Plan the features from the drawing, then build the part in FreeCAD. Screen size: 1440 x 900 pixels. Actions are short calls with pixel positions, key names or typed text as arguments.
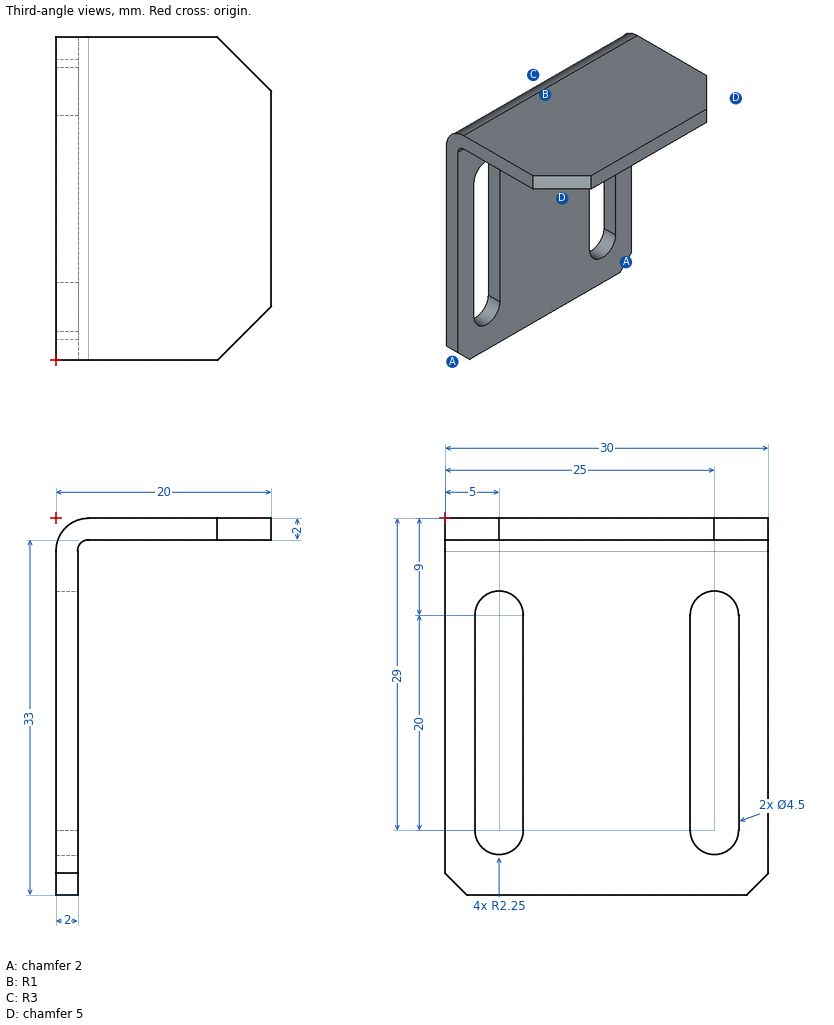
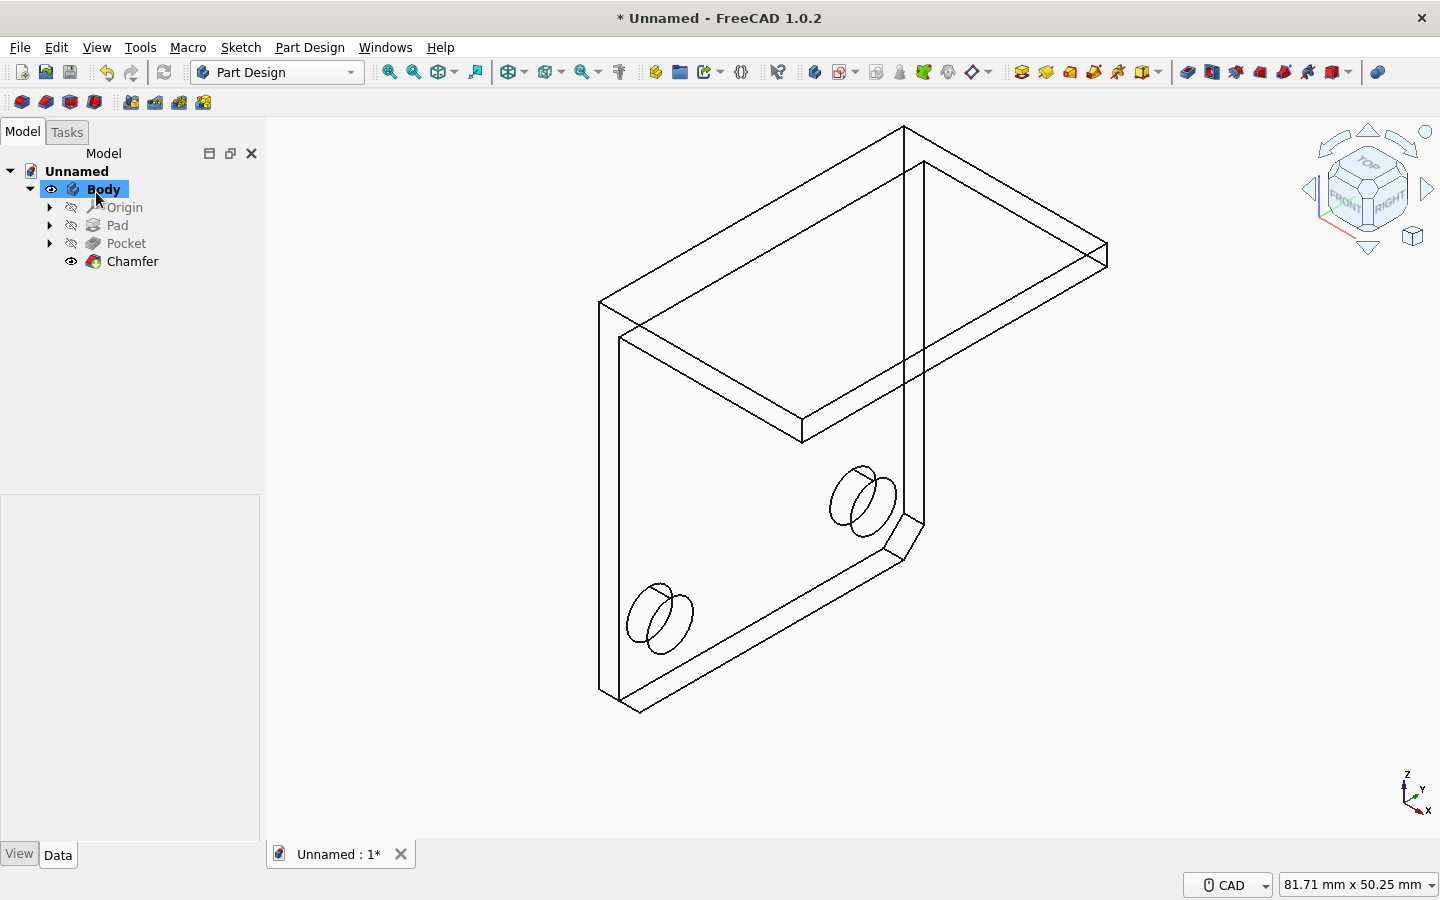
click(772, 248)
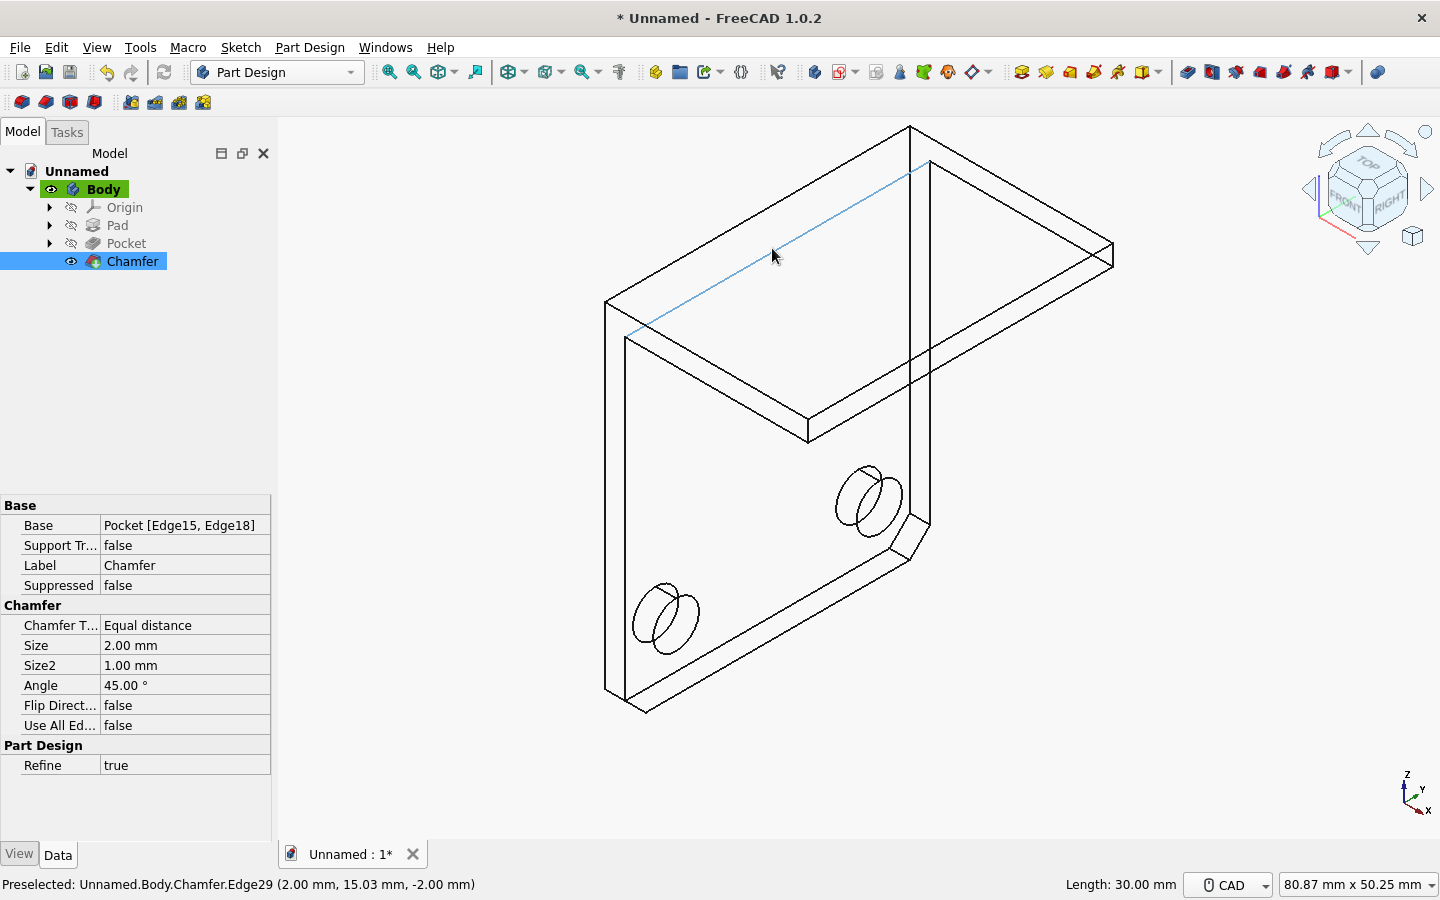
key(v)
key(1)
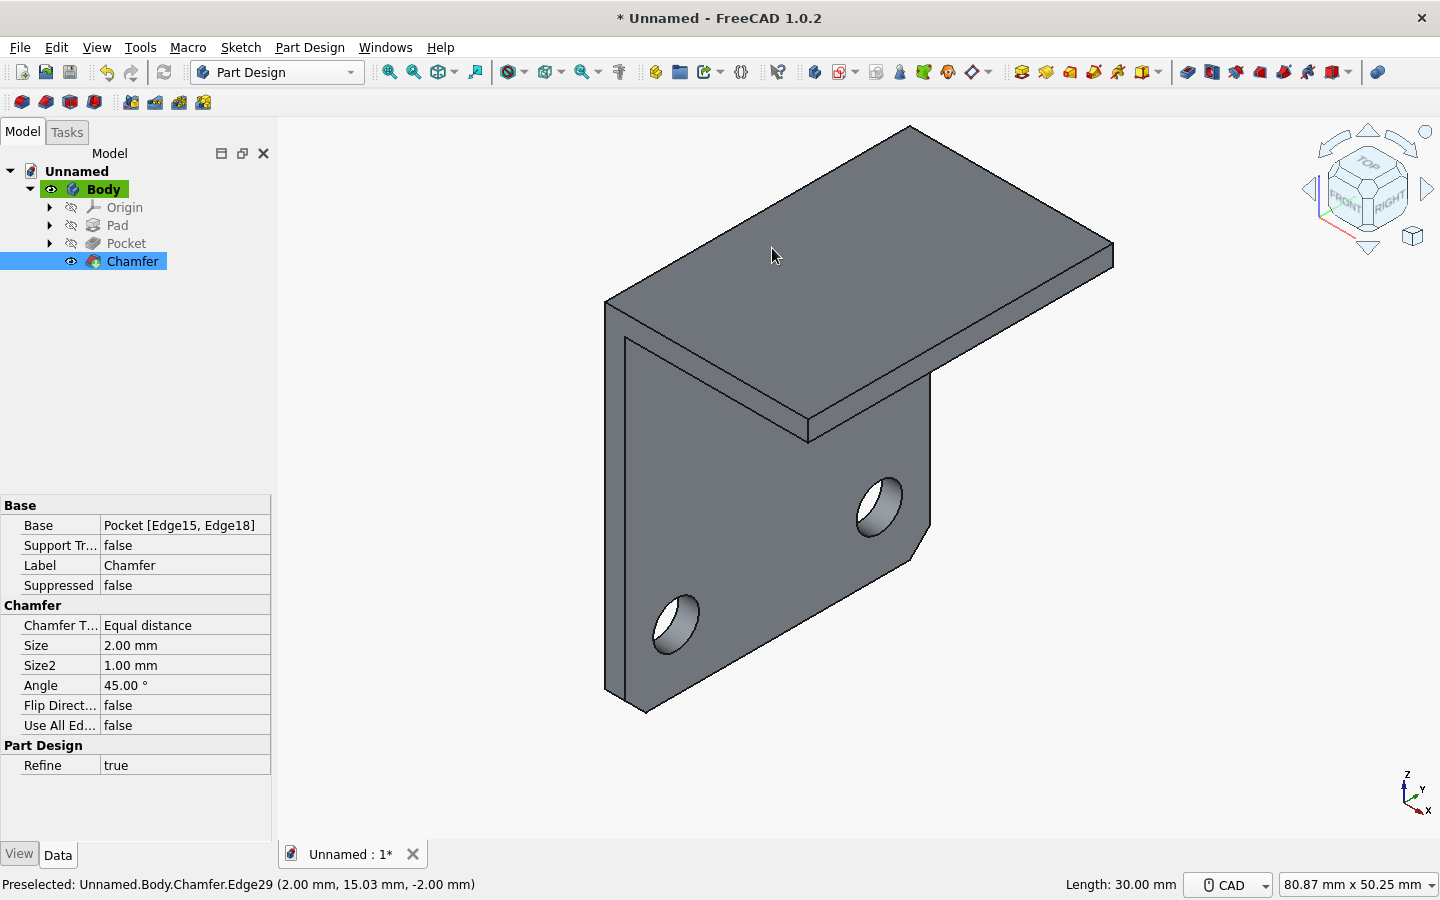
click(22, 102)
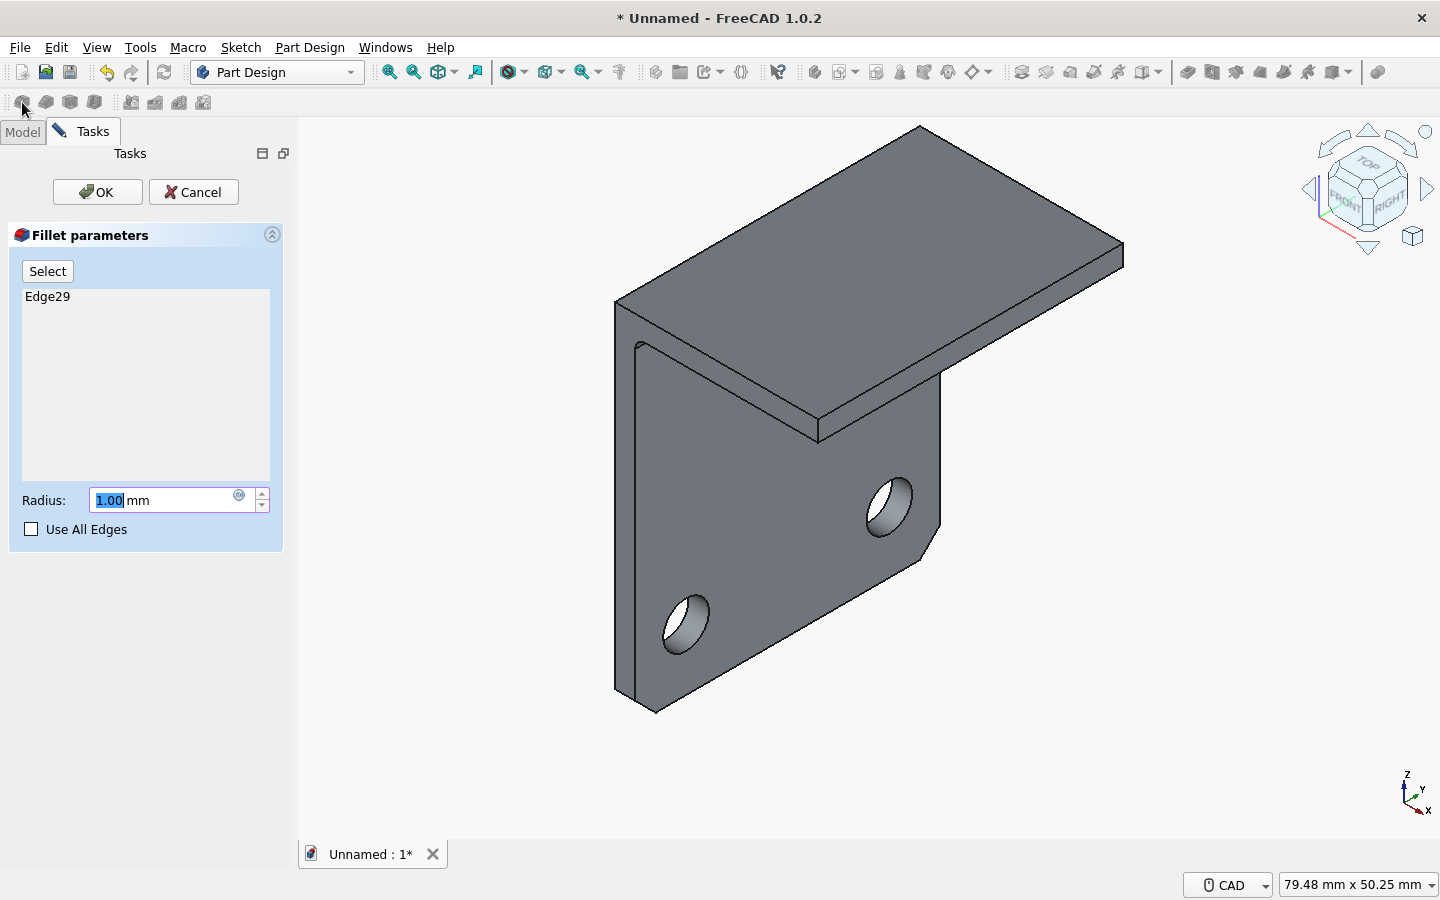
text(1)
key(Tab)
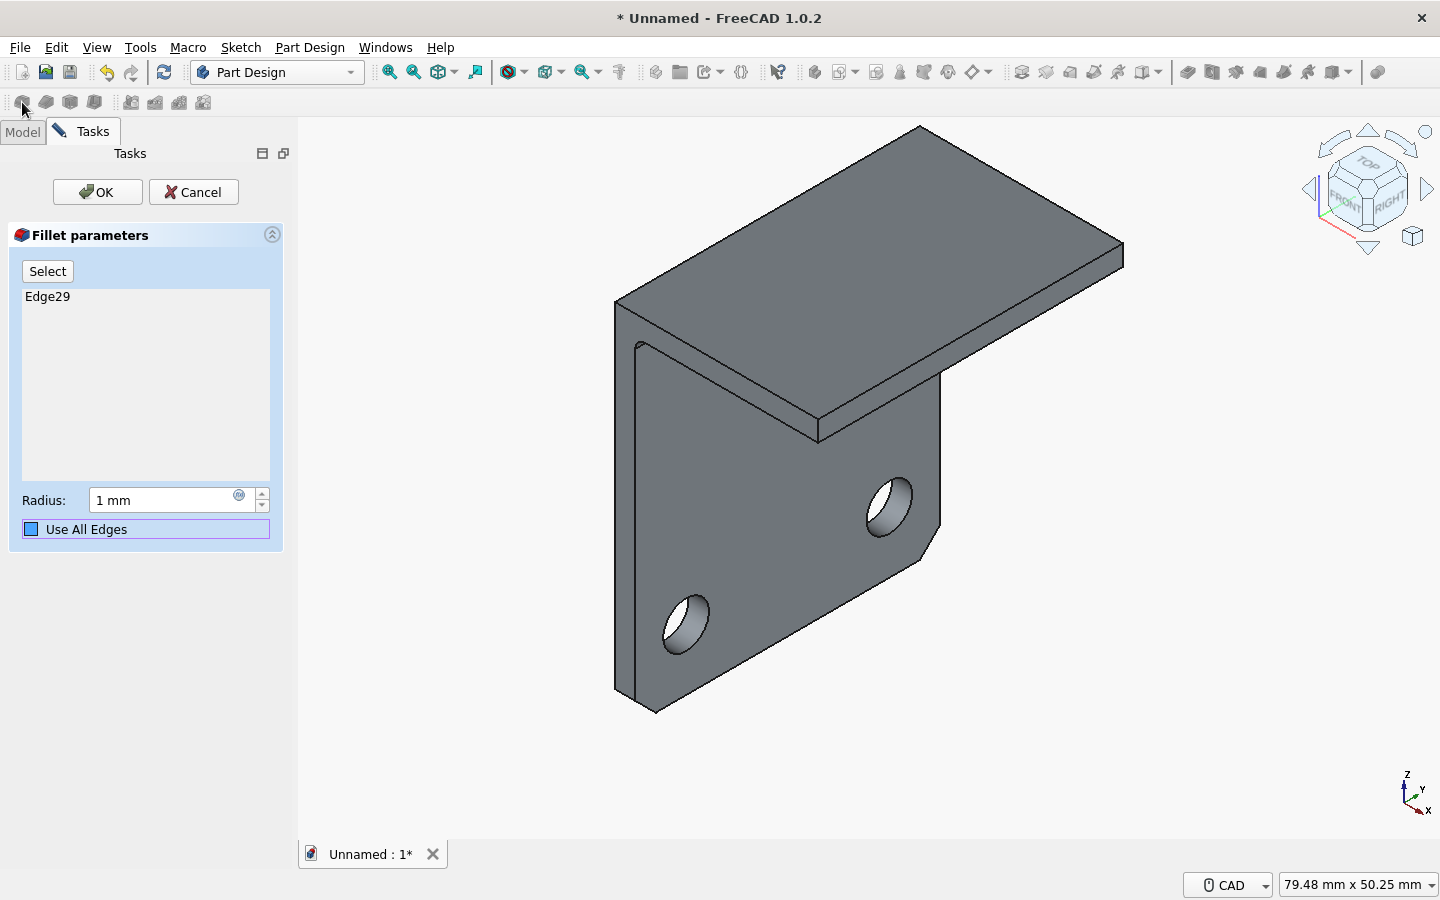
click(98, 192)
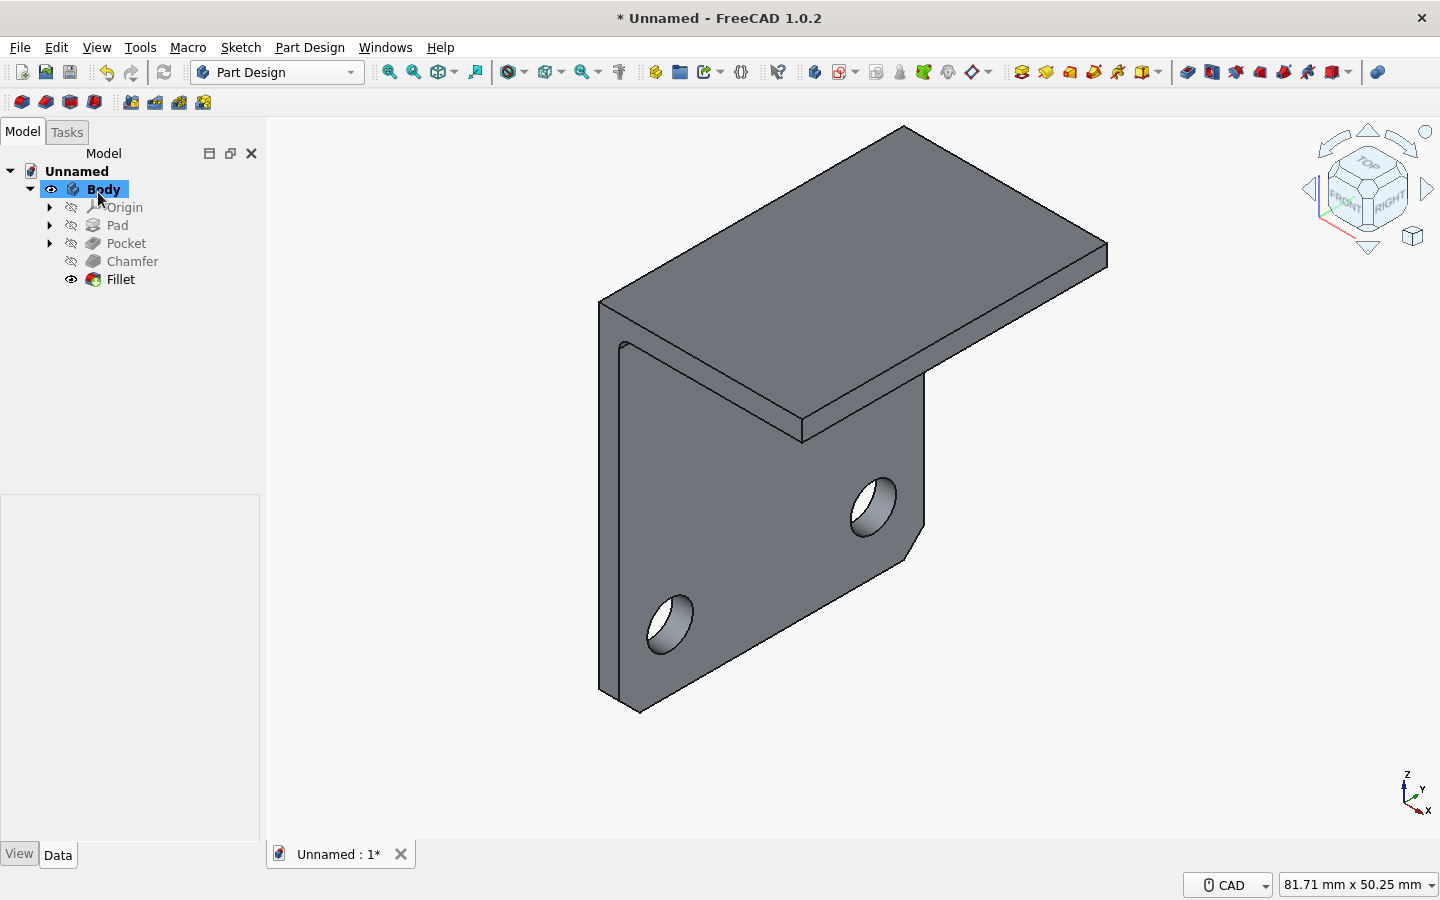
key(2)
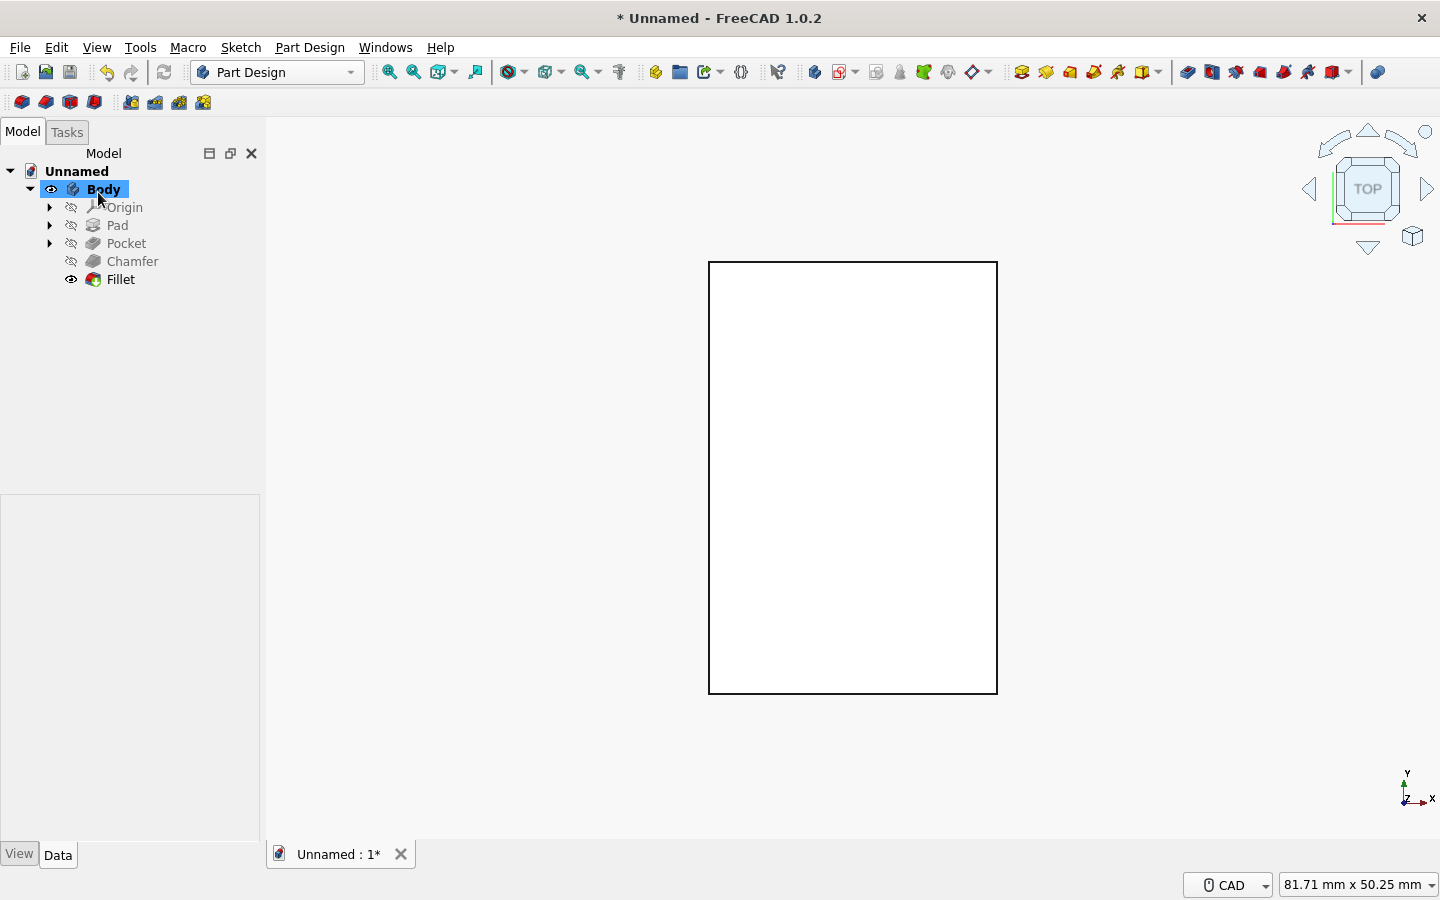
click(709, 434)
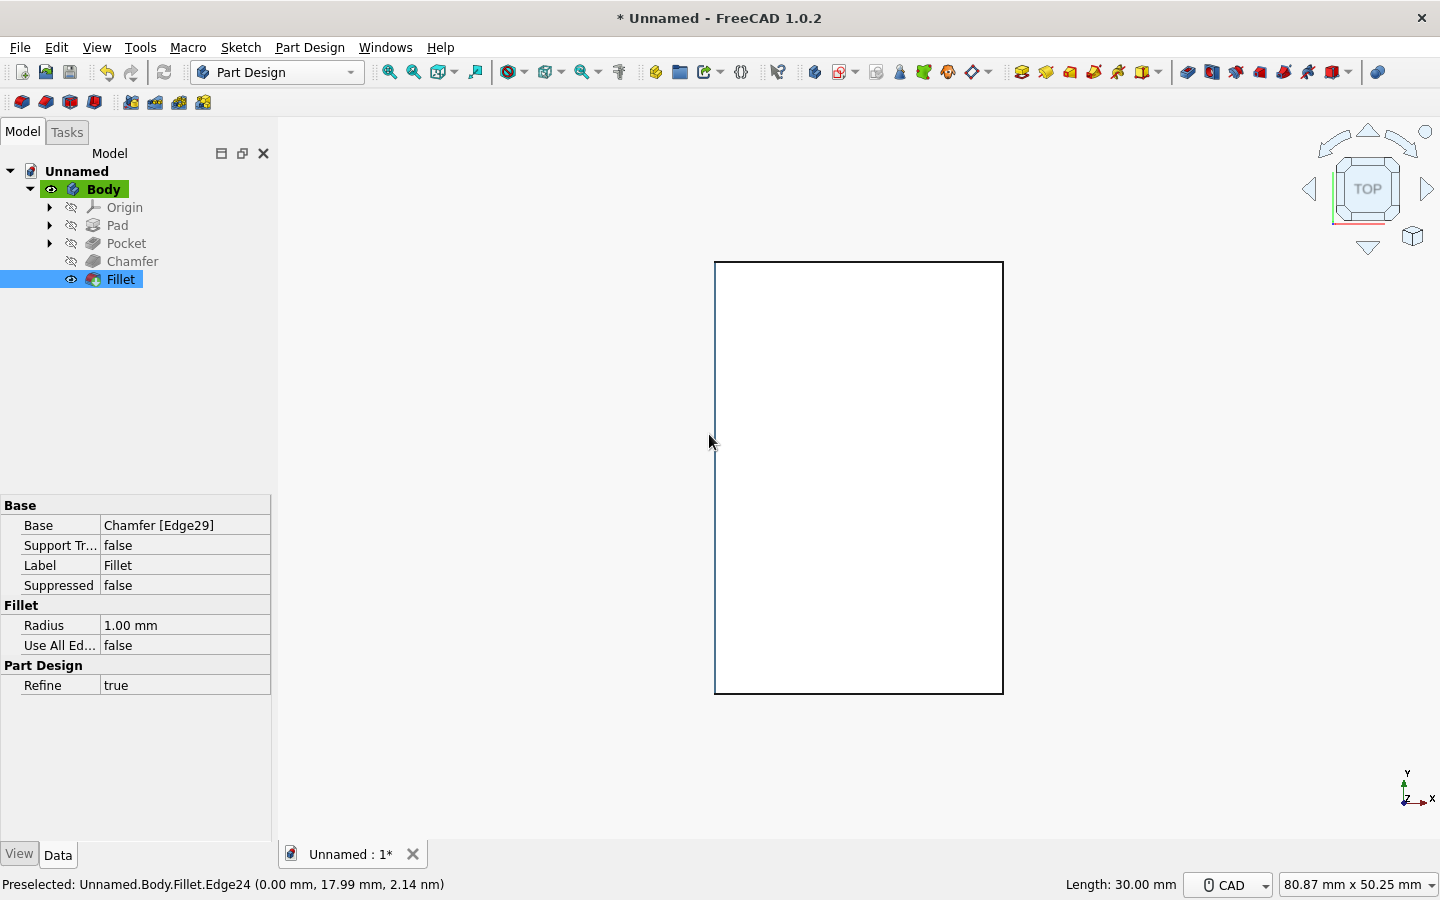
click(22, 102)